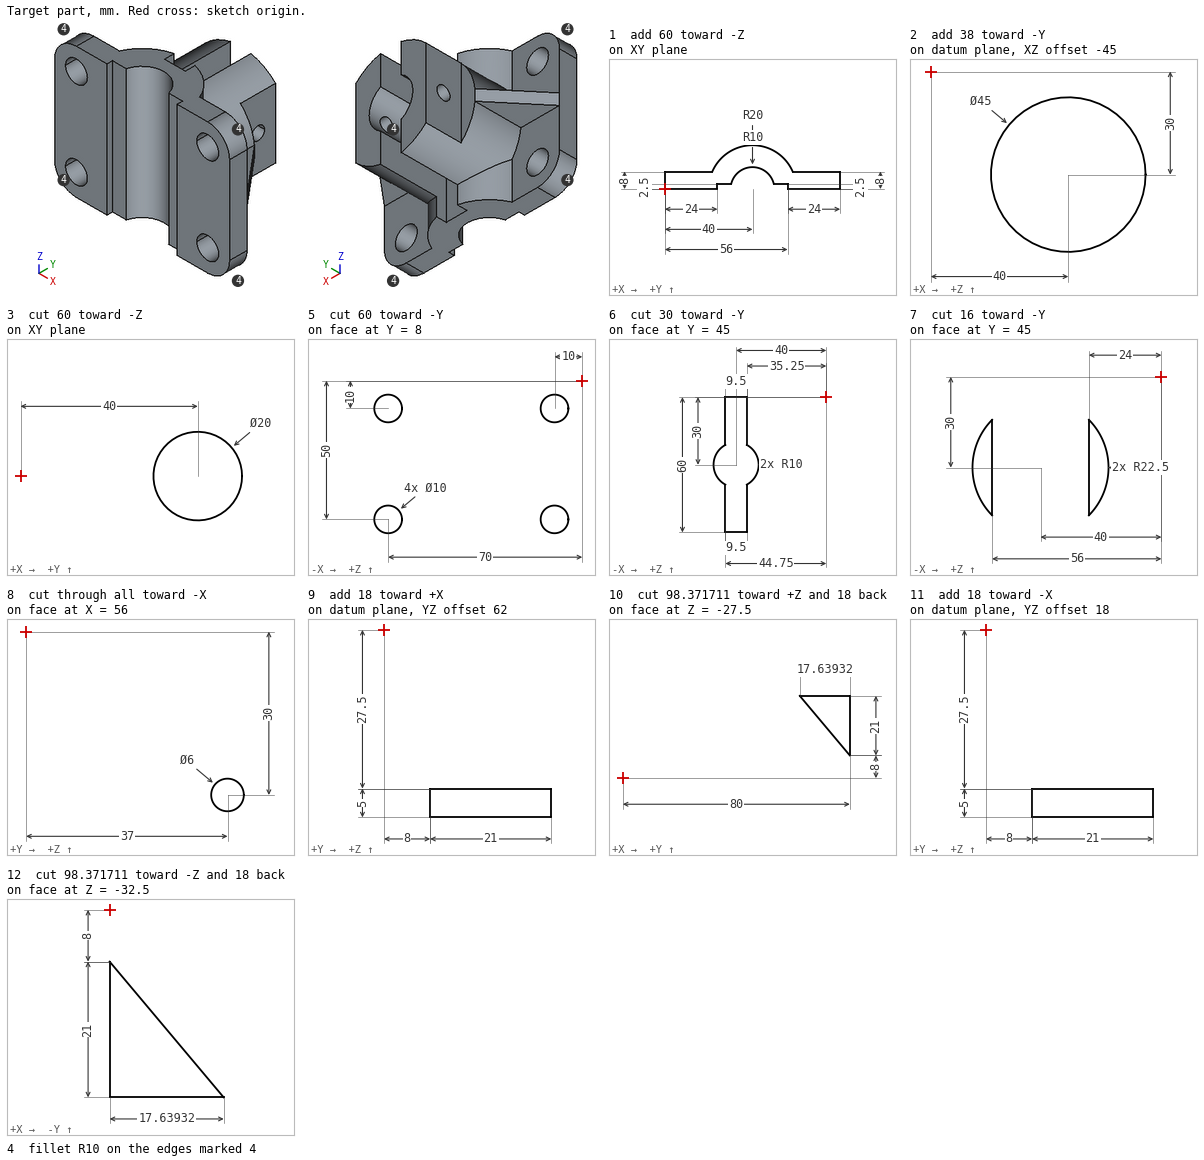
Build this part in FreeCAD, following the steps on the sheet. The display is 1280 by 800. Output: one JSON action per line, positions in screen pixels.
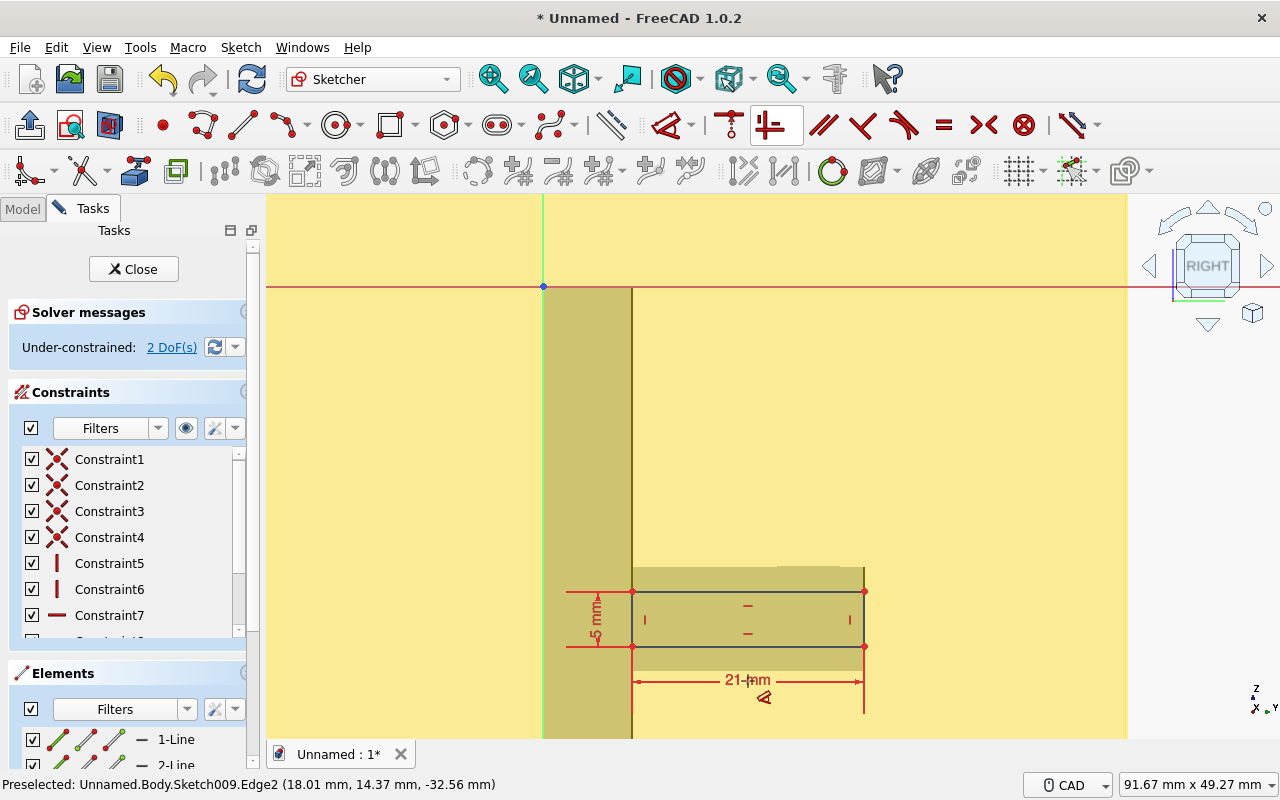
{"action": "left_click", "coordinate": [632, 592]}
{"action": "left_click", "coordinate": [588, 253]}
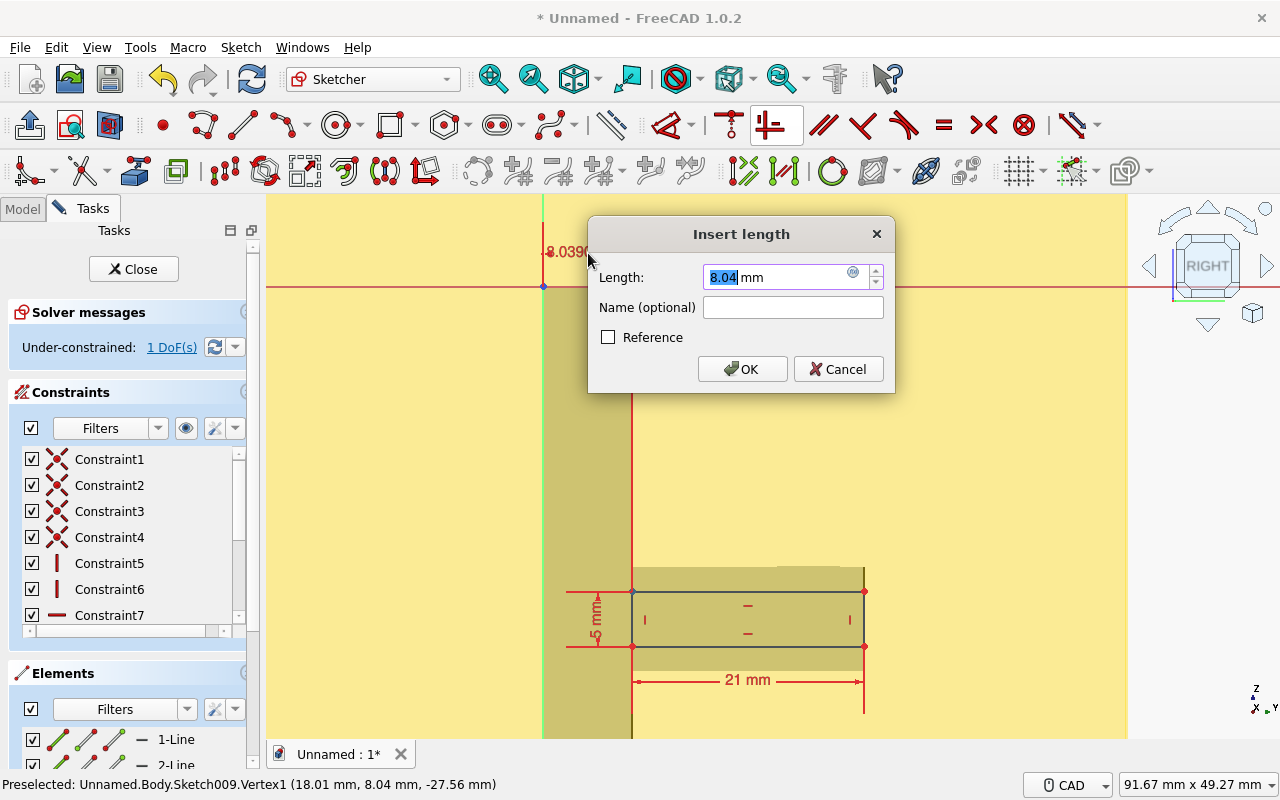
{"action": "type", "text": "8"}
{"action": "key", "text": "Return"}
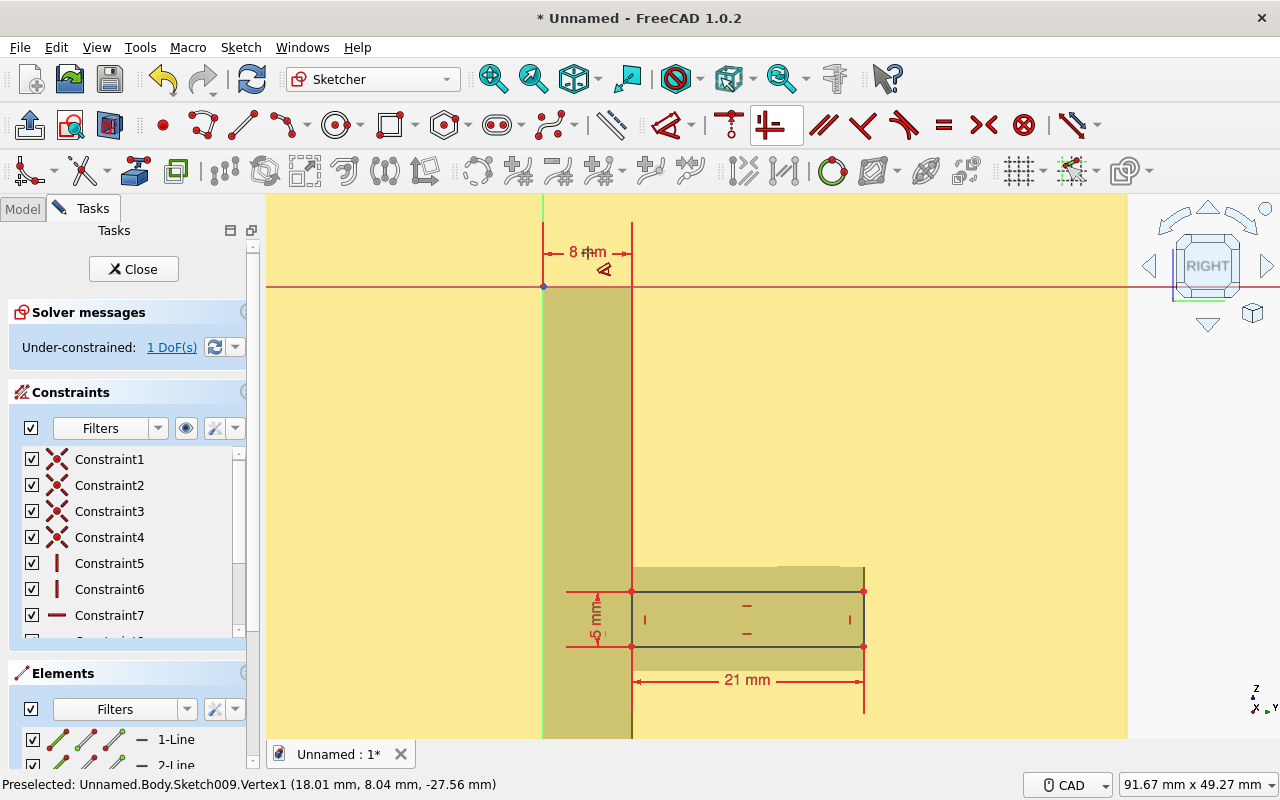
{"action": "left_click", "coordinate": [632, 592]}
{"action": "left_click", "coordinate": [509, 439]}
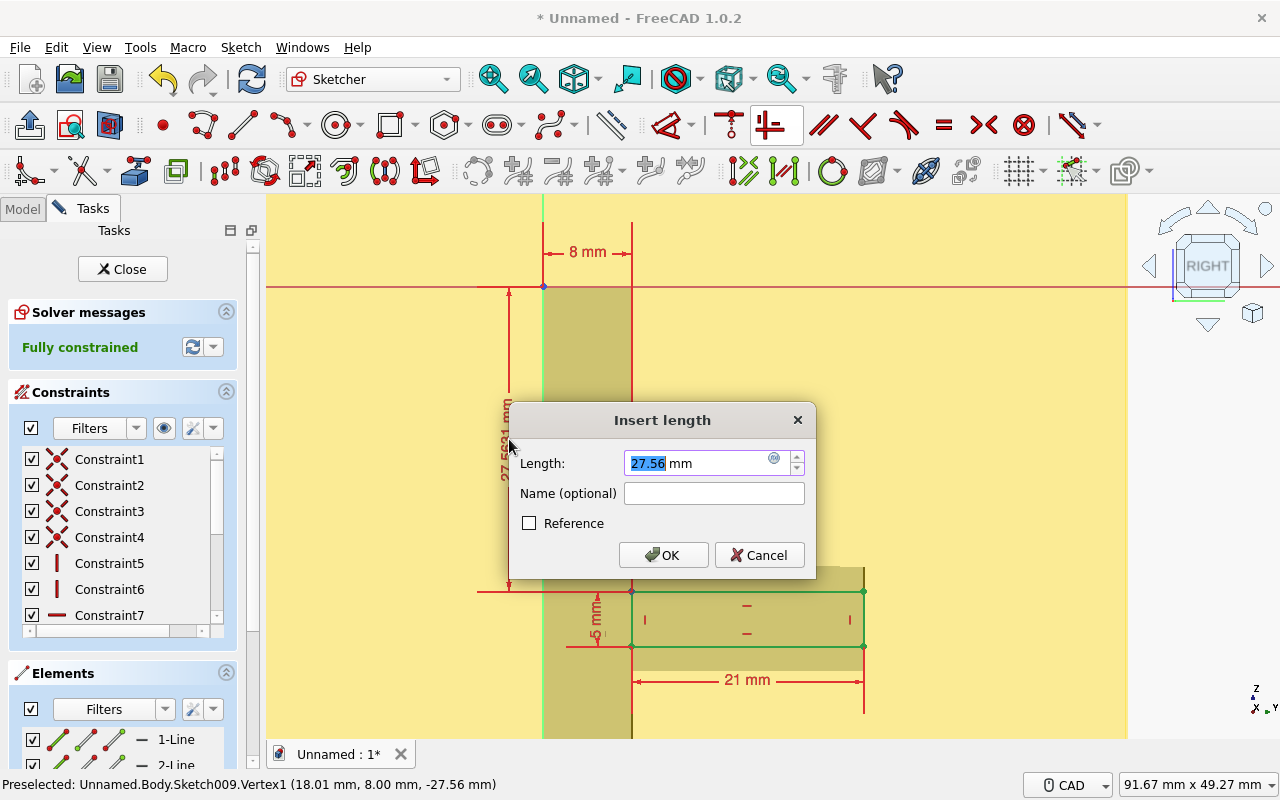
{"action": "type", "text": "27.5"}
{"action": "key", "text": "Return"}
{"action": "key", "text": "Escape"}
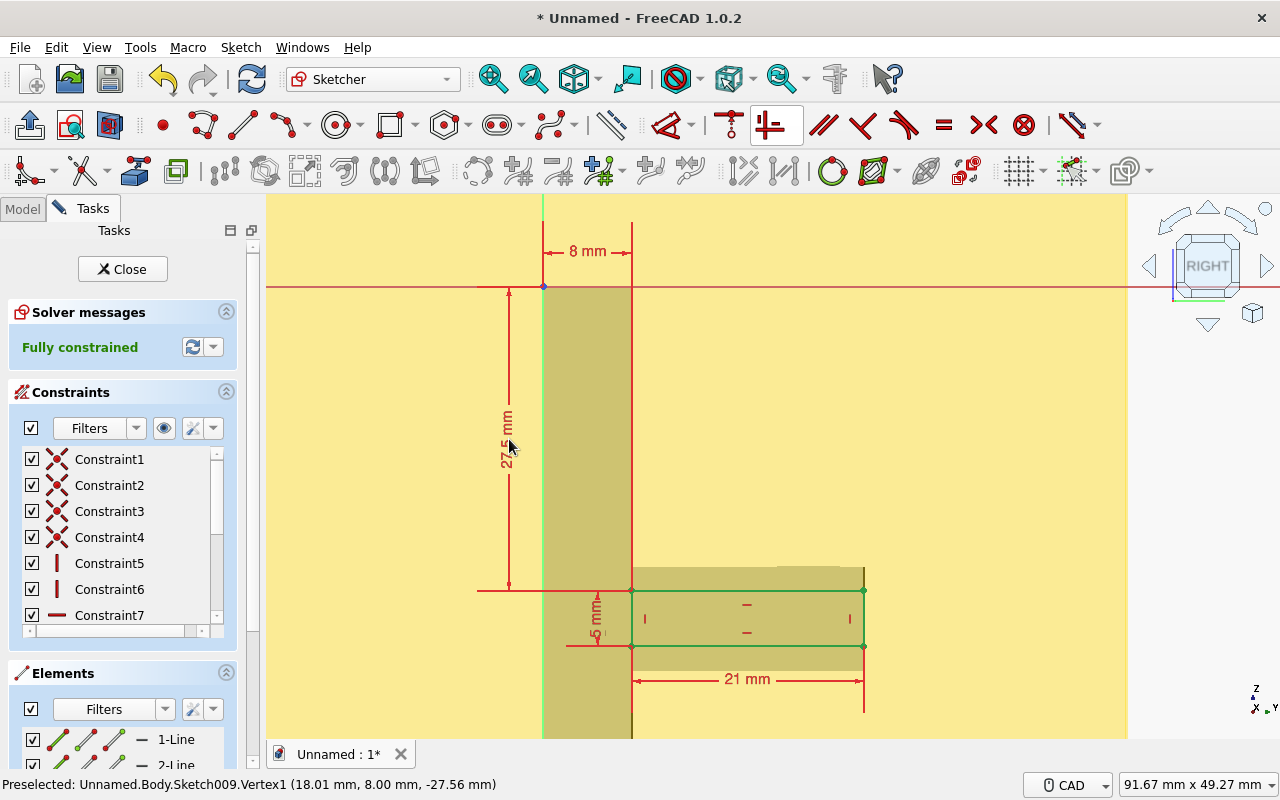
{"action": "left_click", "coordinate": [123, 269]}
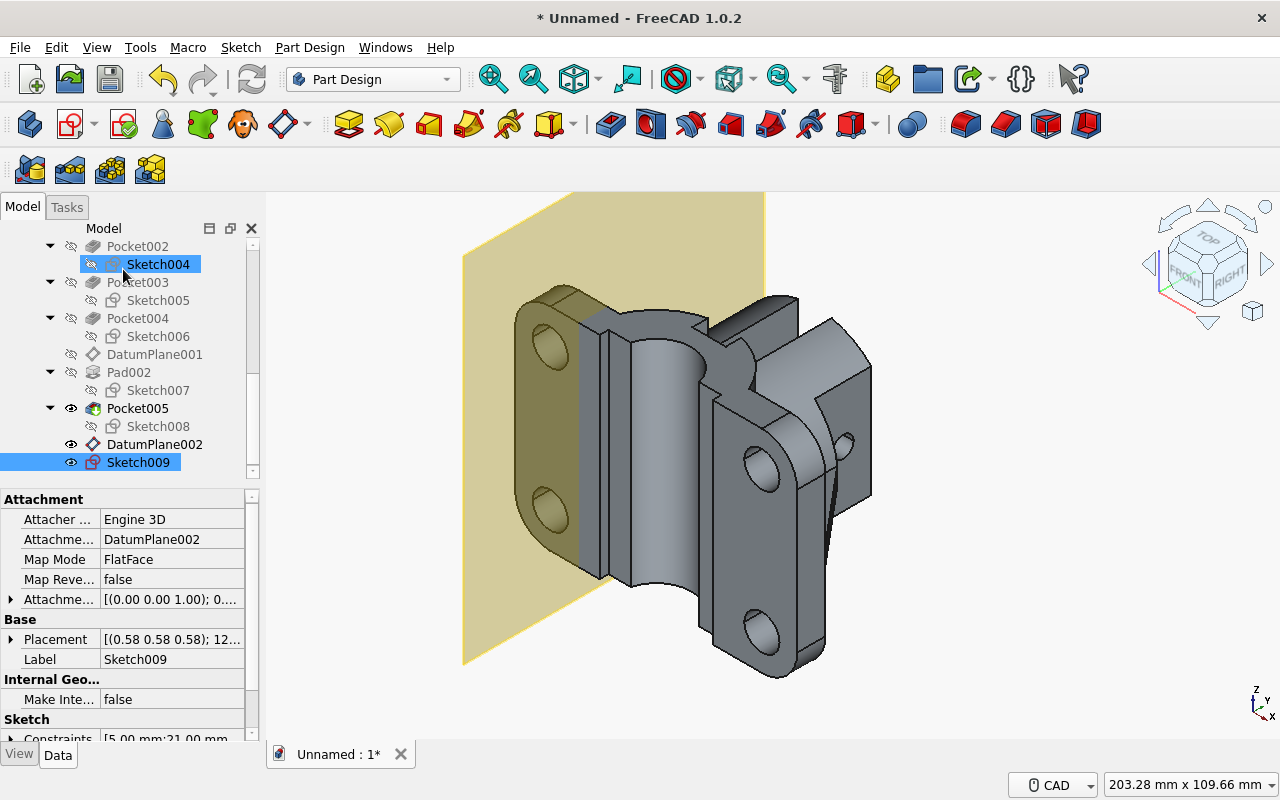
{"action": "left_click", "coordinate": [350, 124]}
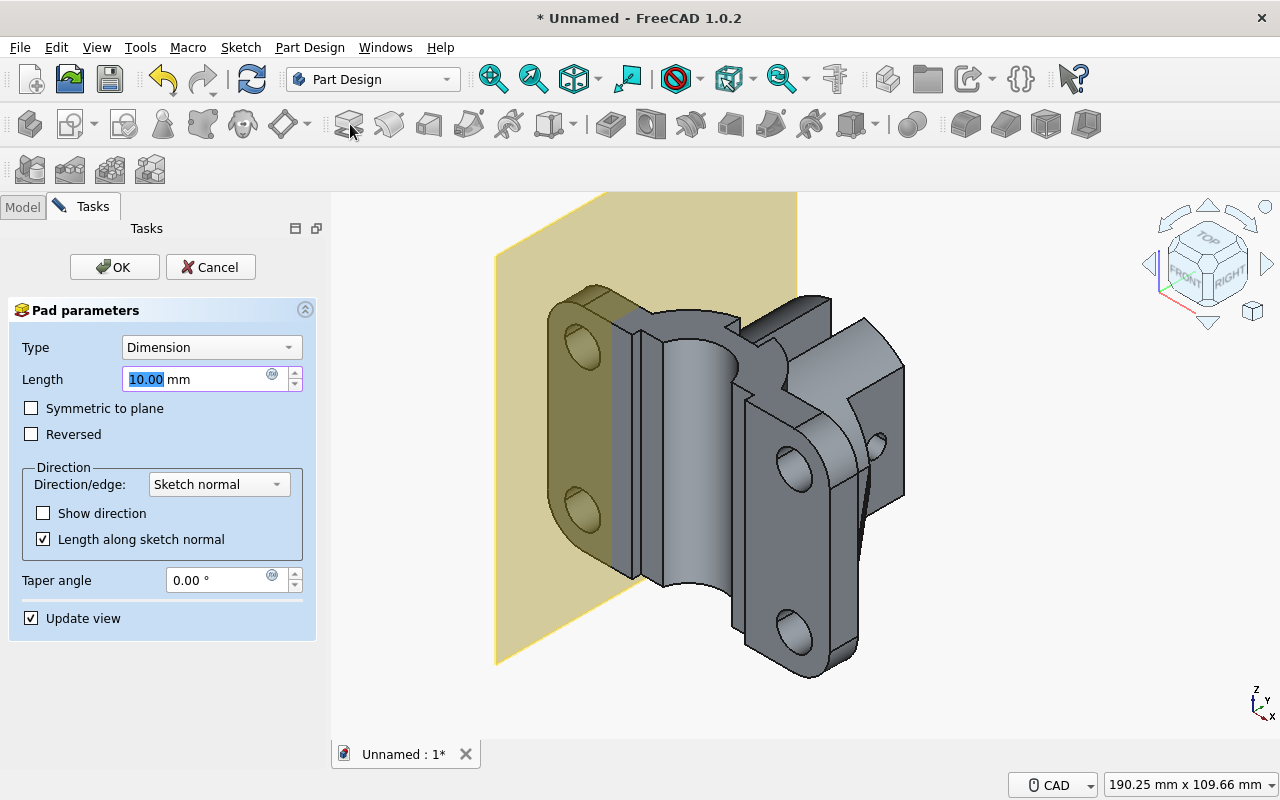
{"action": "type", "text": "18"}
{"action": "key", "text": "Tab"}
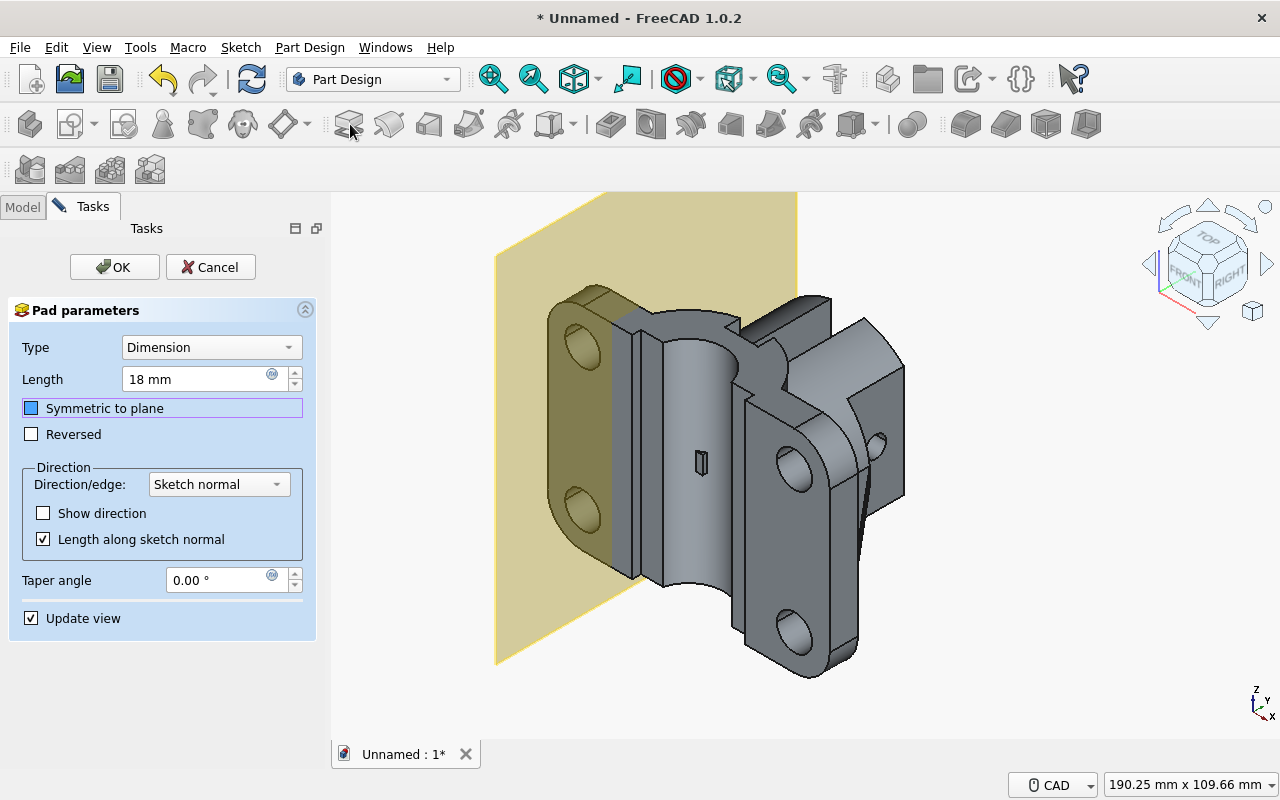
{"action": "left_click", "coordinate": [30, 434]}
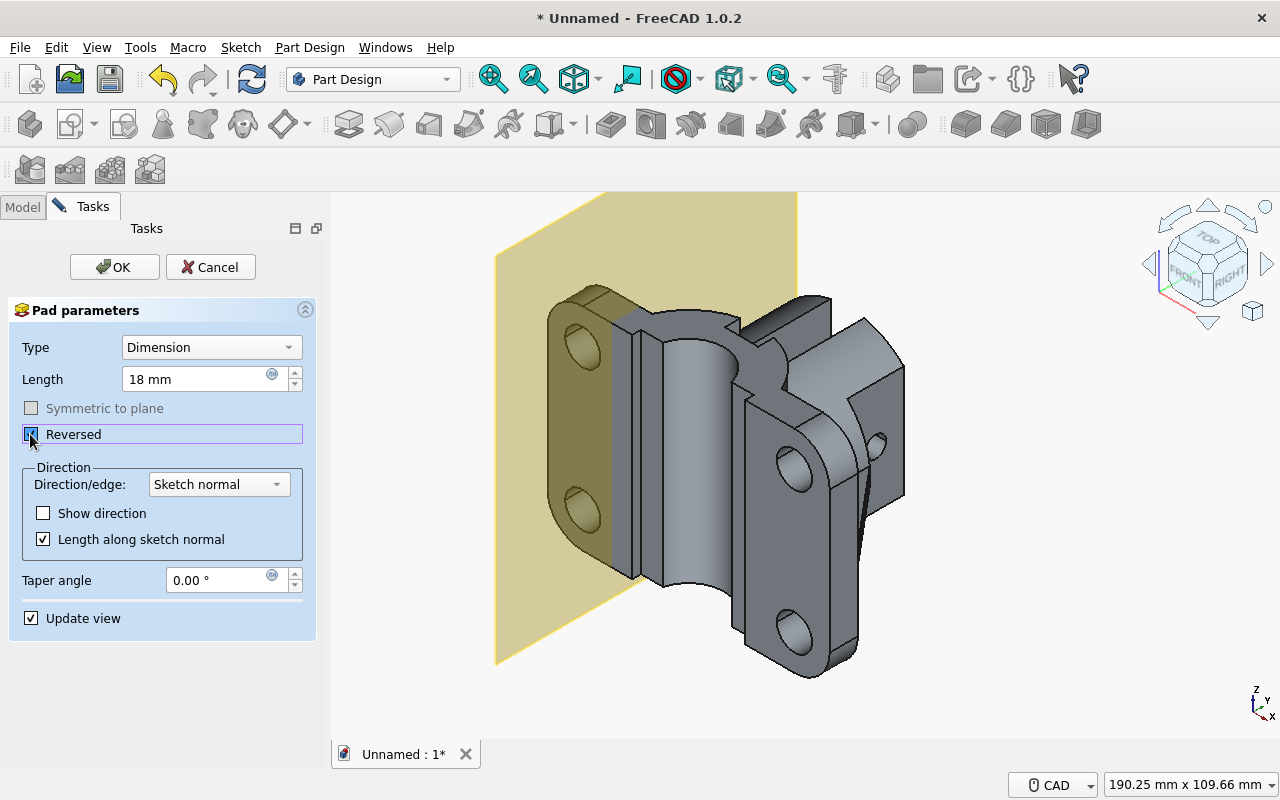
{"action": "left_click", "coordinate": [115, 267]}